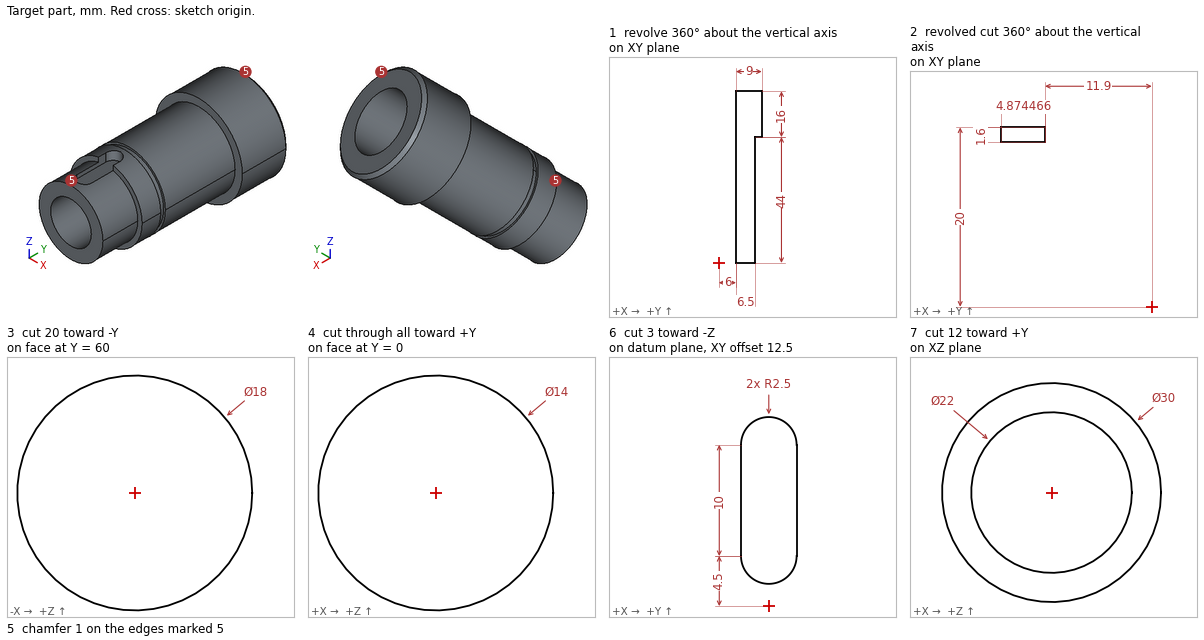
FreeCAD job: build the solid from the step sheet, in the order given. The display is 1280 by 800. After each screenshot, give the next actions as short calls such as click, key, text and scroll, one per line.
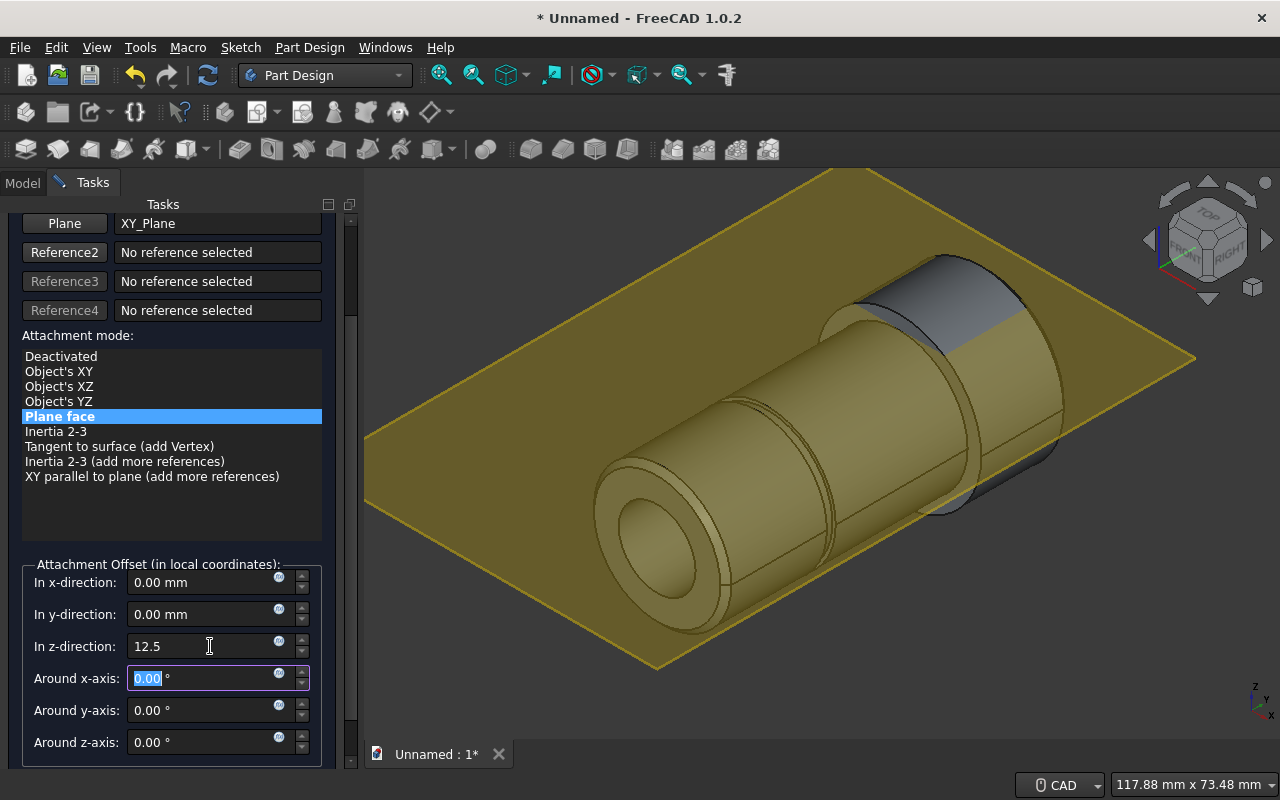
scroll(351, 491, up, 3)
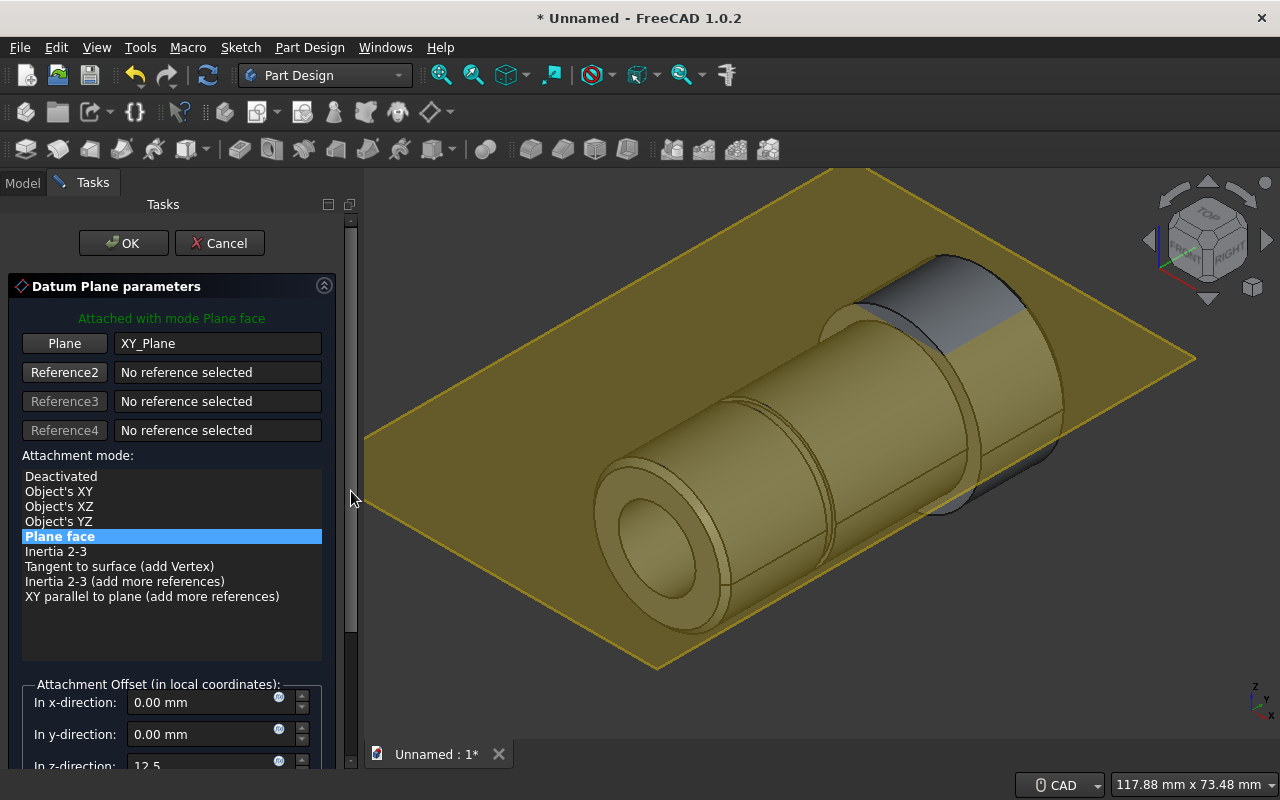
click(124, 243)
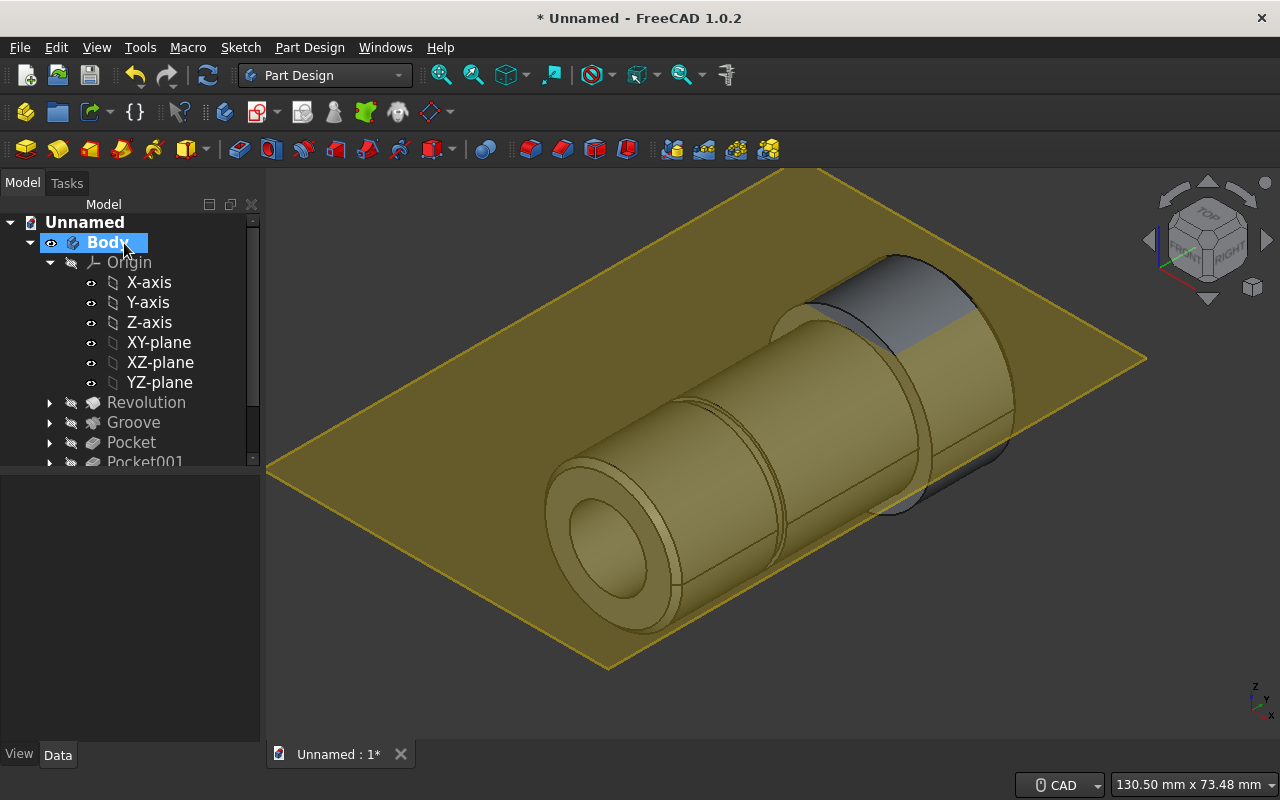
scroll(100, 338, down, 3)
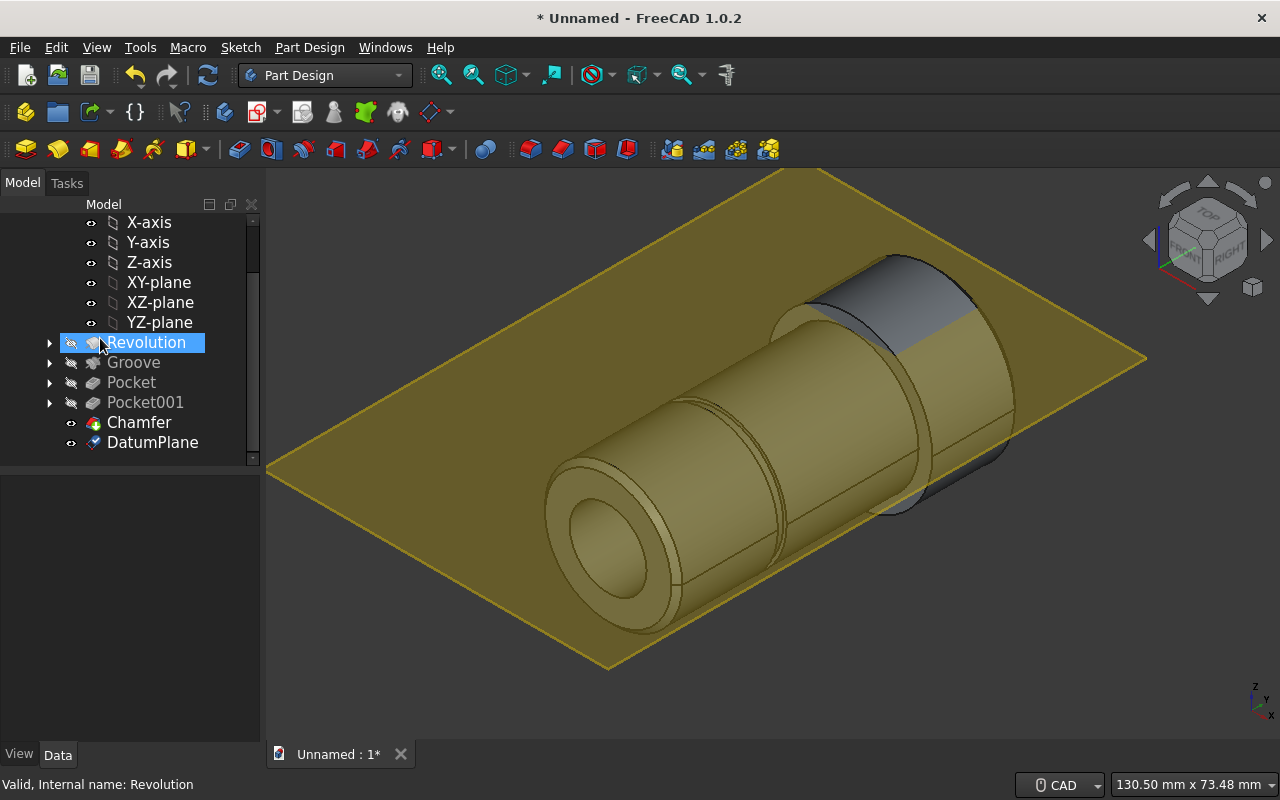
click(116, 443)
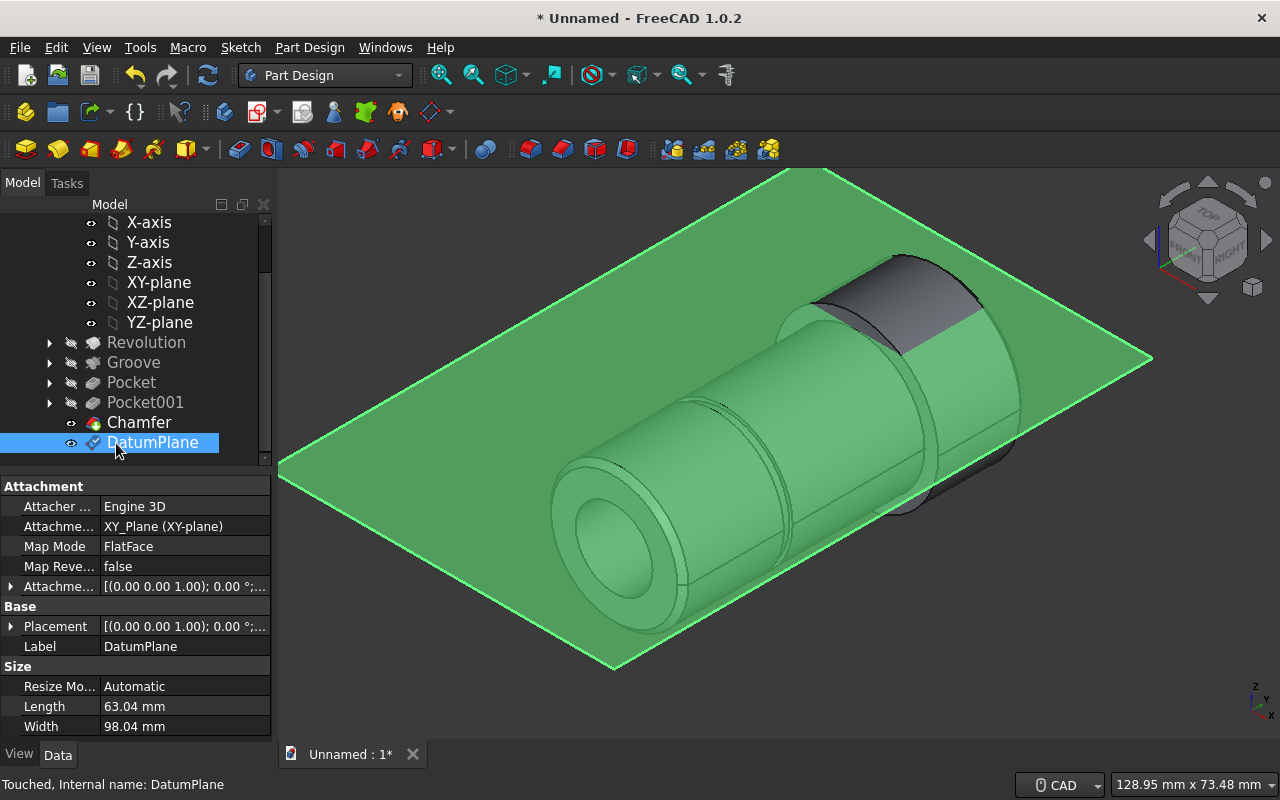
click(258, 112)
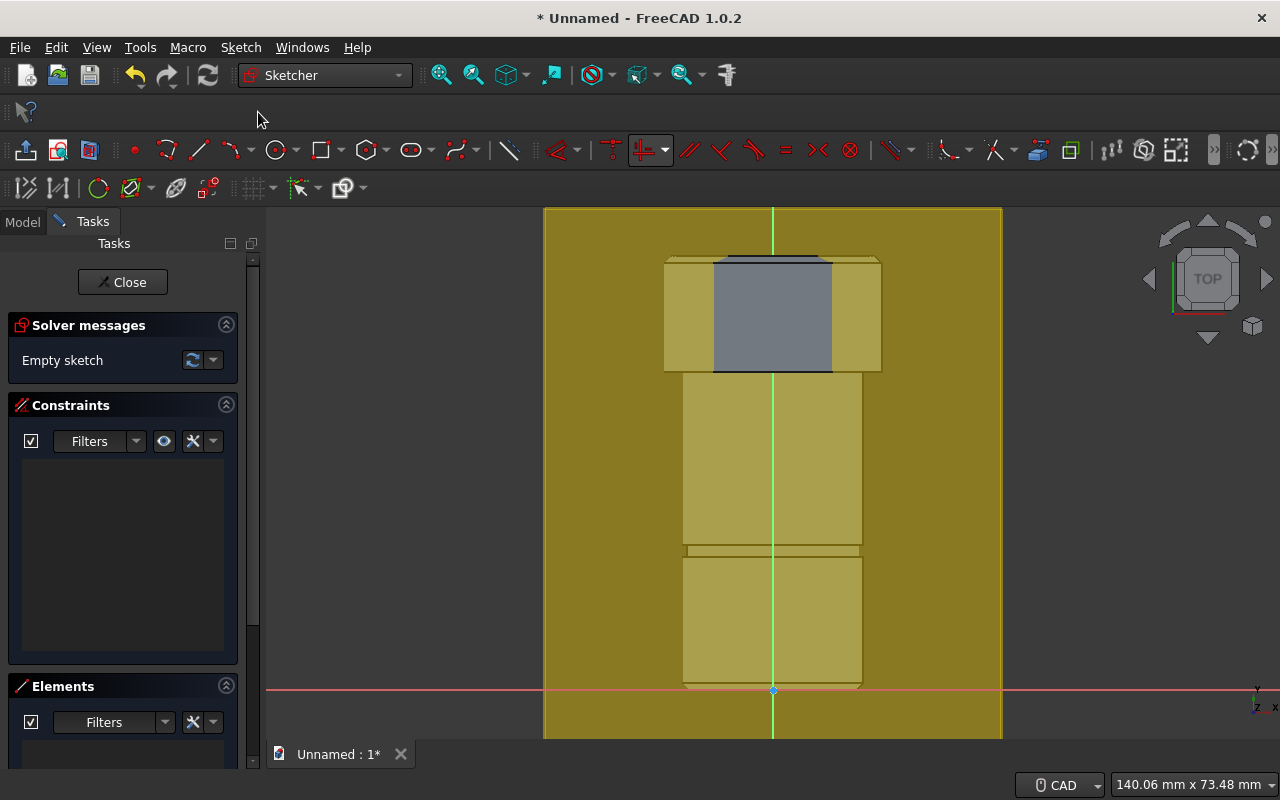
click(90, 150)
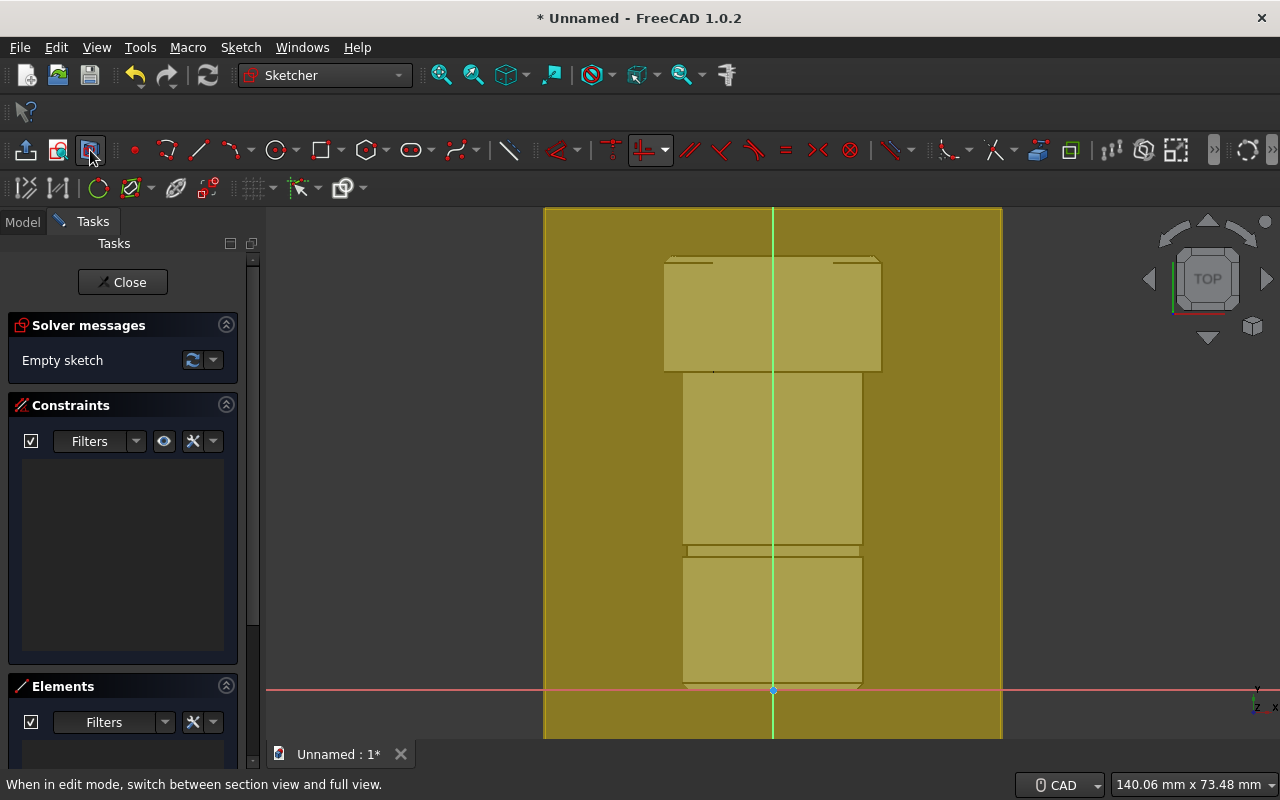
scroll(813, 711, up, 5)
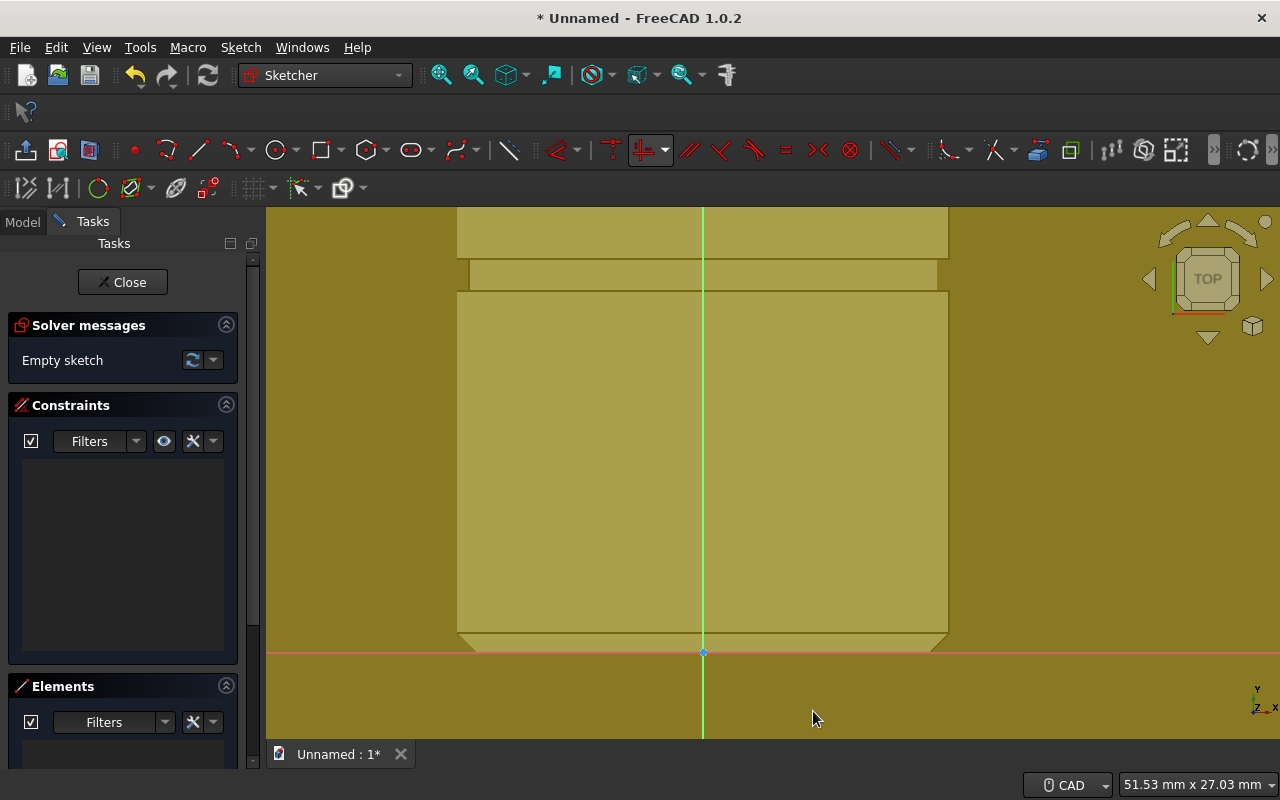
click(412, 150)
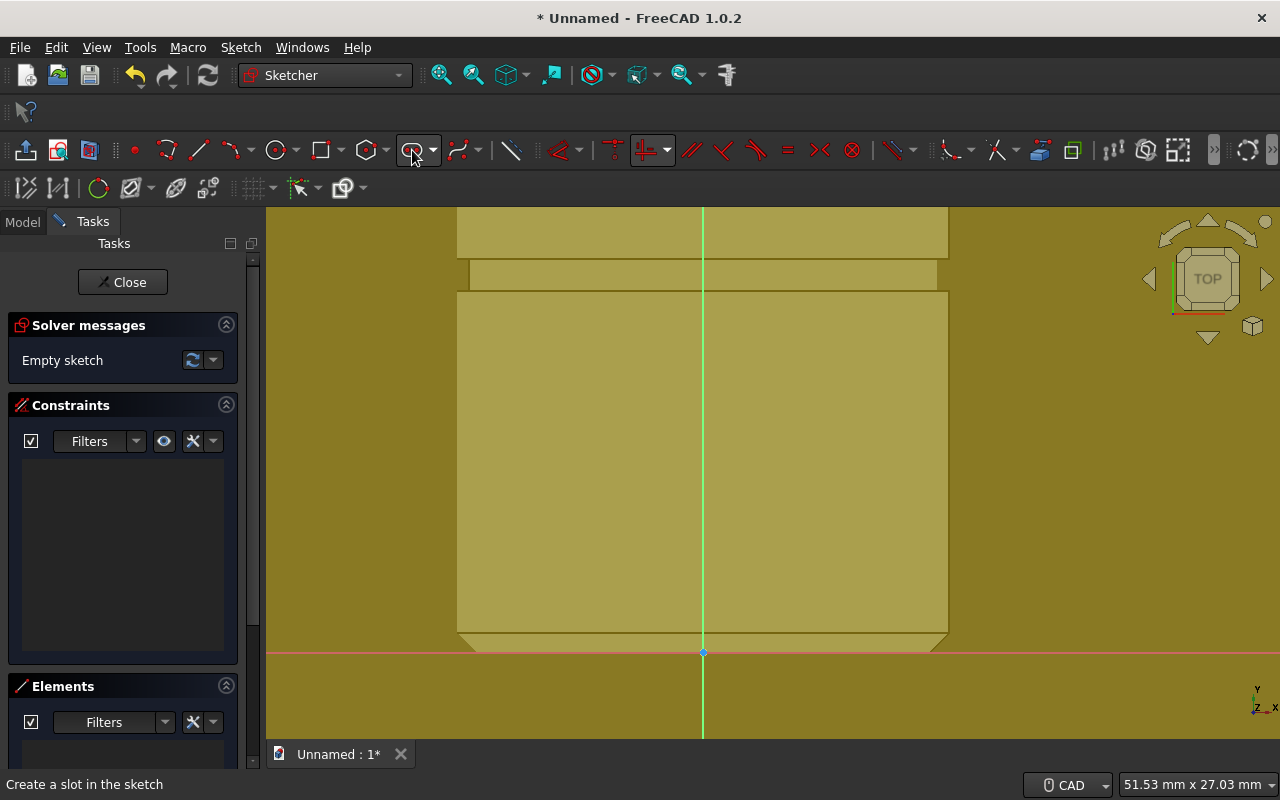
click(703, 564)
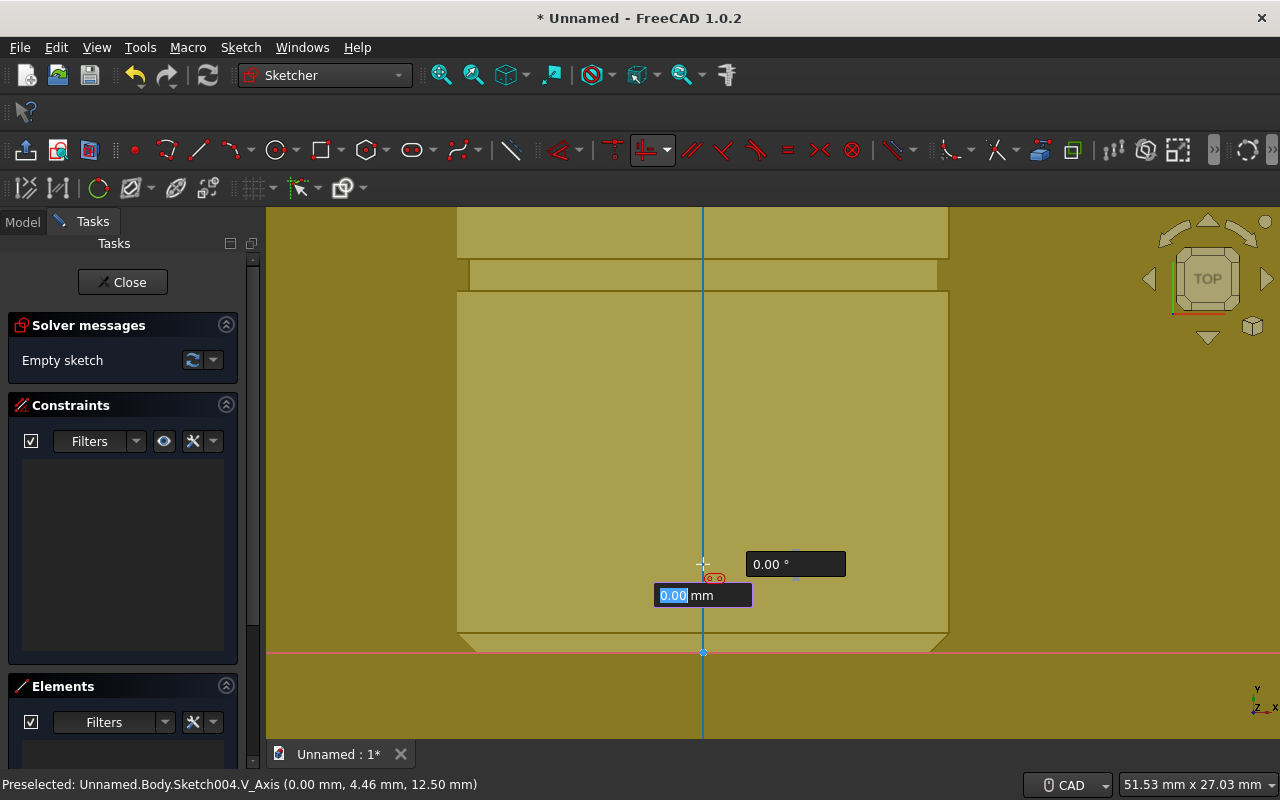
click(712, 367)